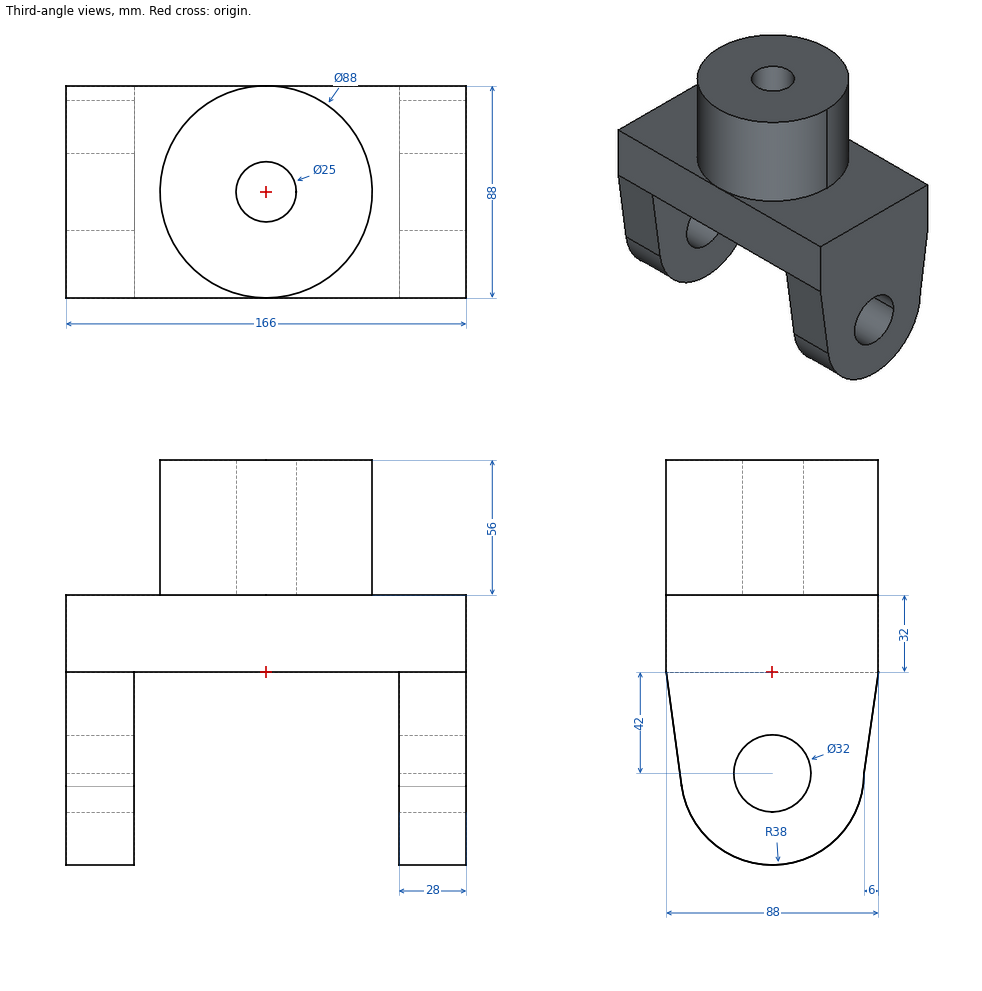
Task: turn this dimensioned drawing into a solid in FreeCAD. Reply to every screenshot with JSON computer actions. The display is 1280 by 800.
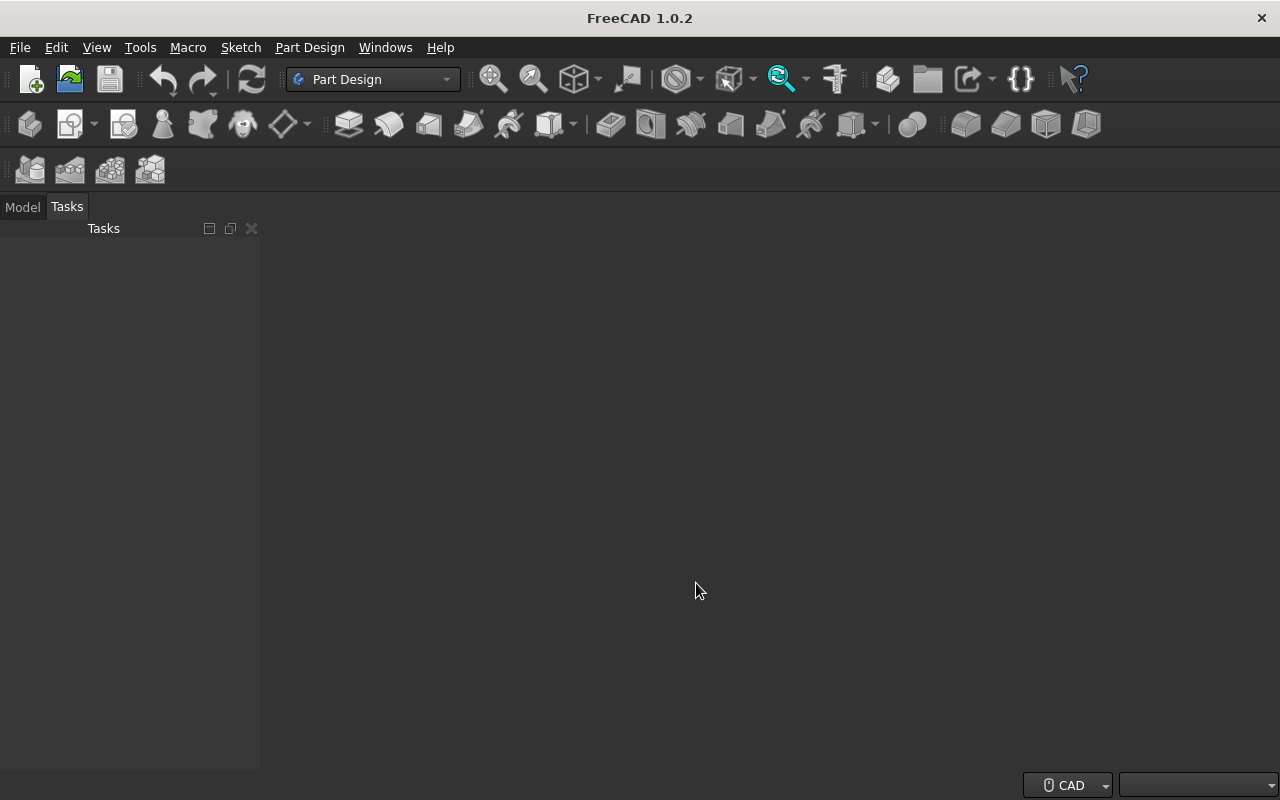
{"action": "left_click", "coordinate": [30, 80]}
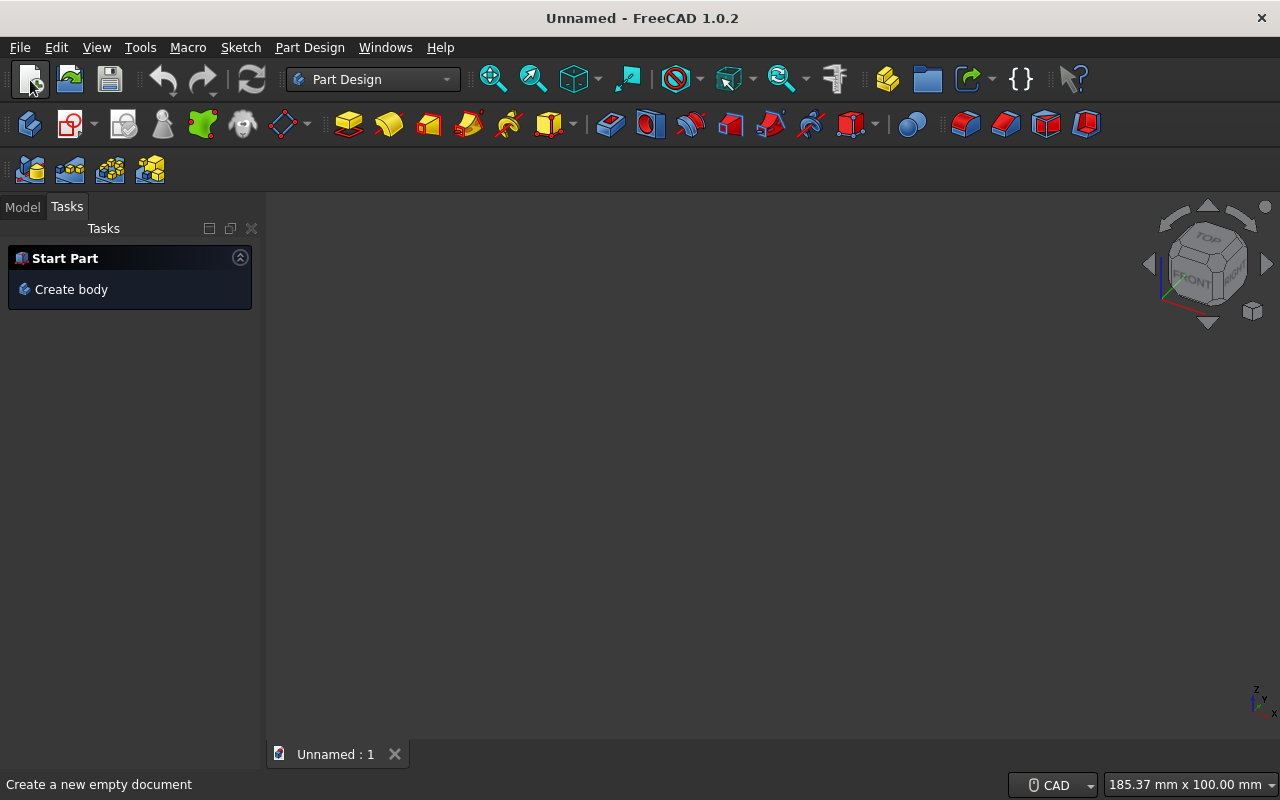
{"action": "left_click", "coordinate": [70, 124]}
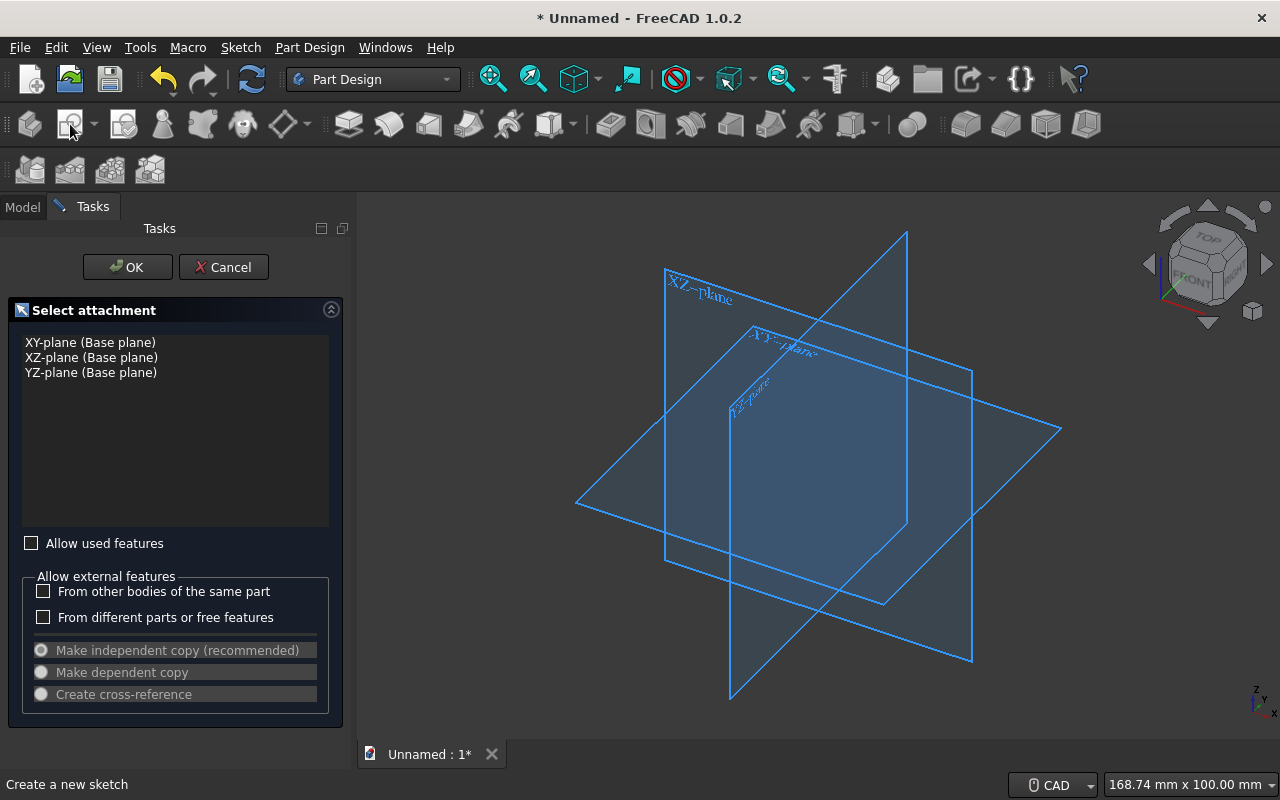
{"action": "left_click", "coordinate": [82, 342]}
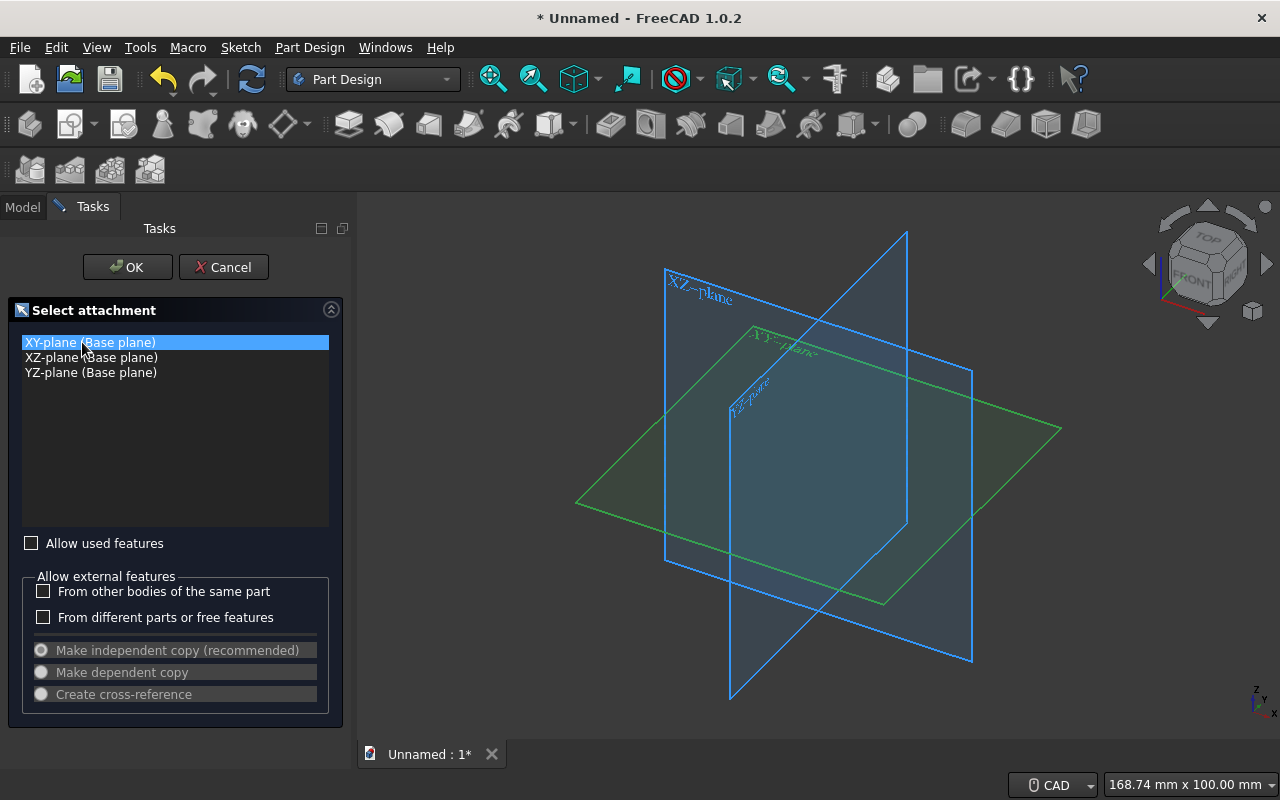
{"action": "left_click", "coordinate": [128, 267]}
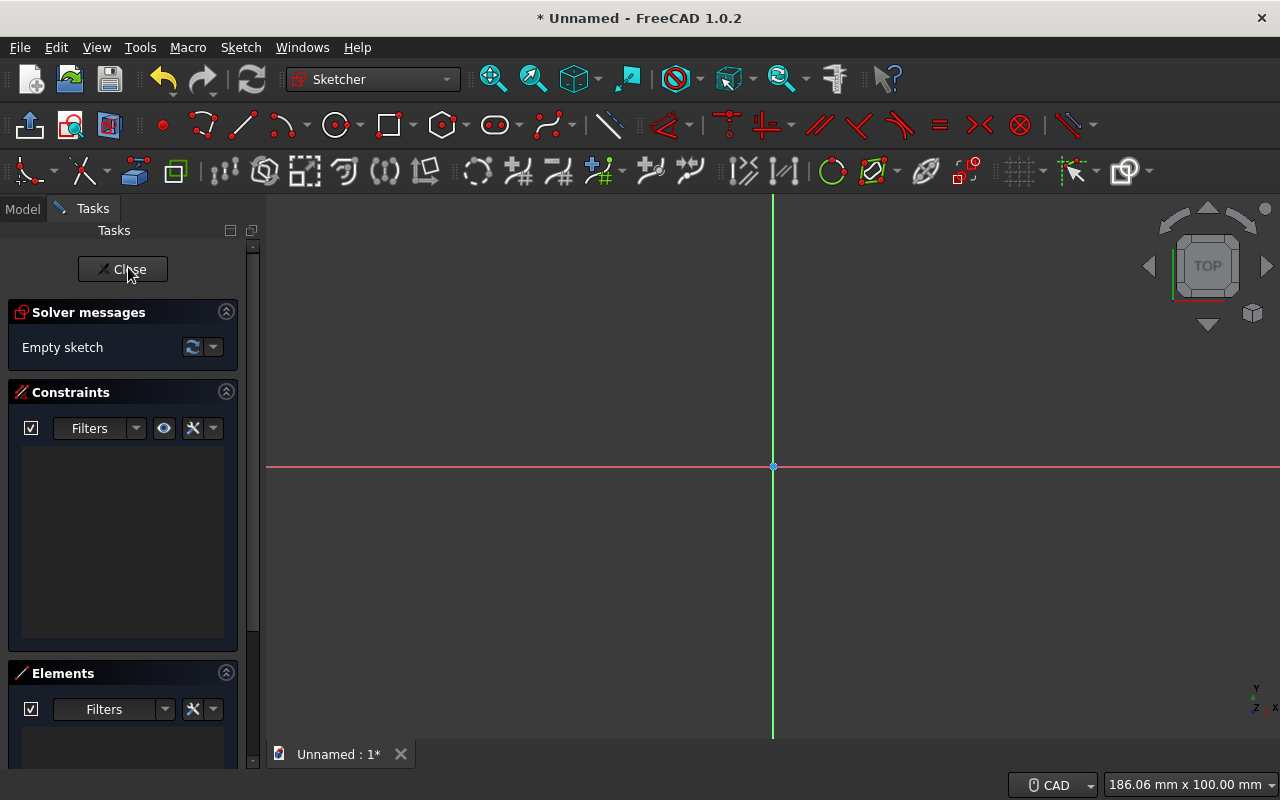
{"action": "scroll", "coordinate": [565, 466], "scroll_direction": "down", "scroll_amount": 2}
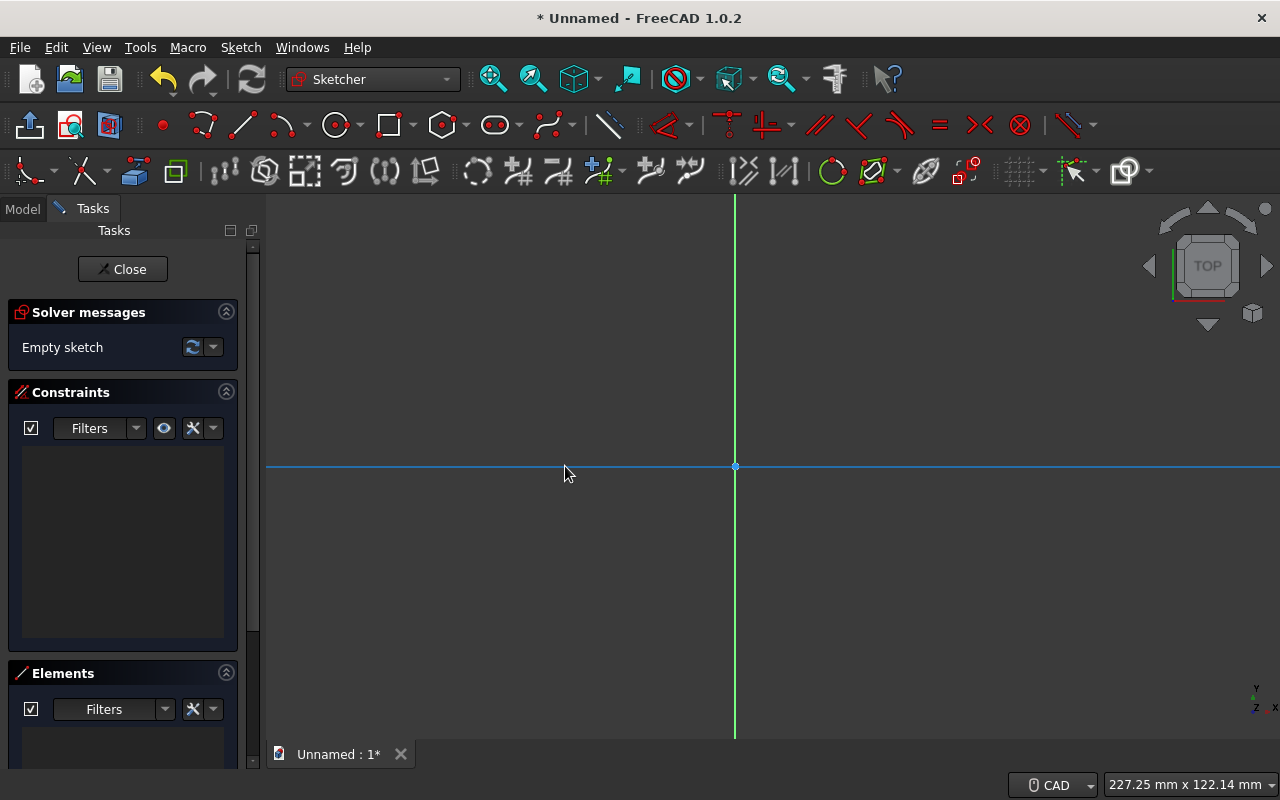
{"action": "key", "text": "g v"}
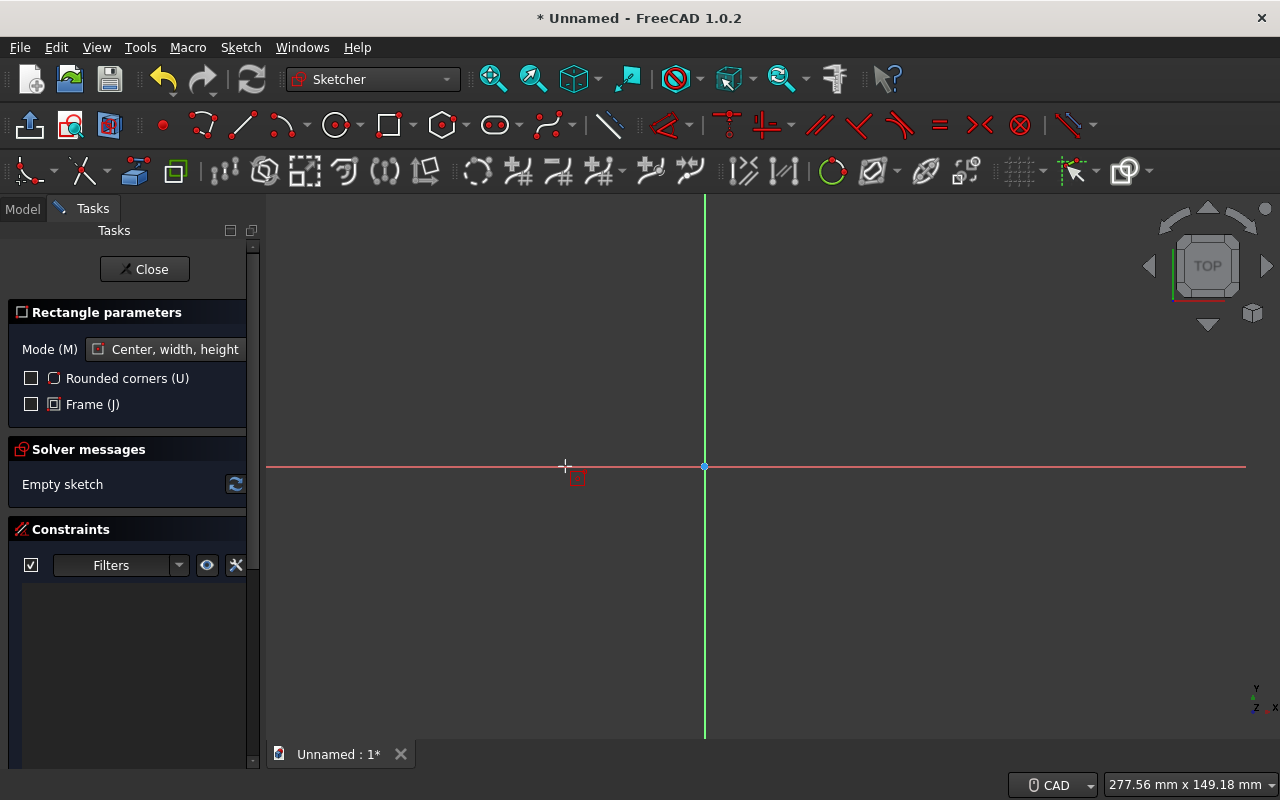
{"action": "left_click", "coordinate": [705, 466]}
{"action": "left_click", "coordinate": [1008, 306]}
{"action": "key", "text": "Escape"}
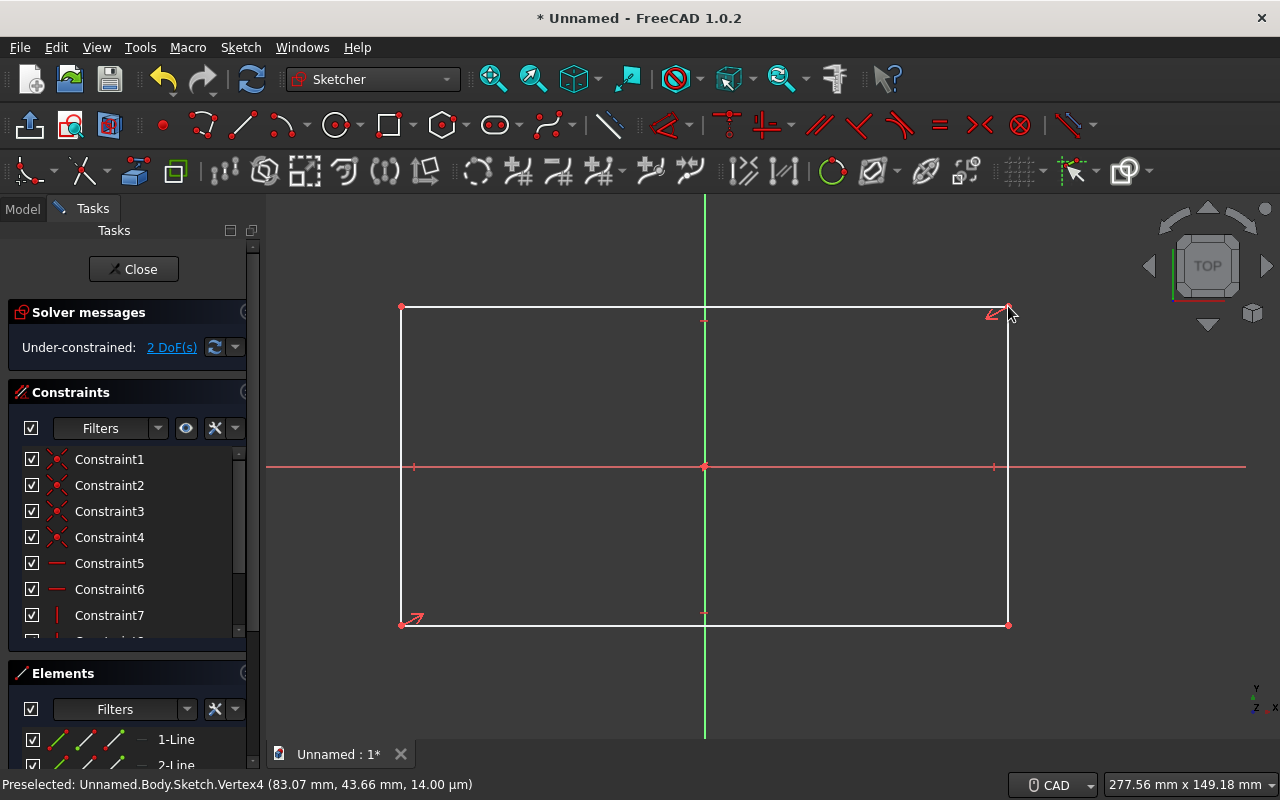
{"action": "left_click", "coordinate": [664, 126]}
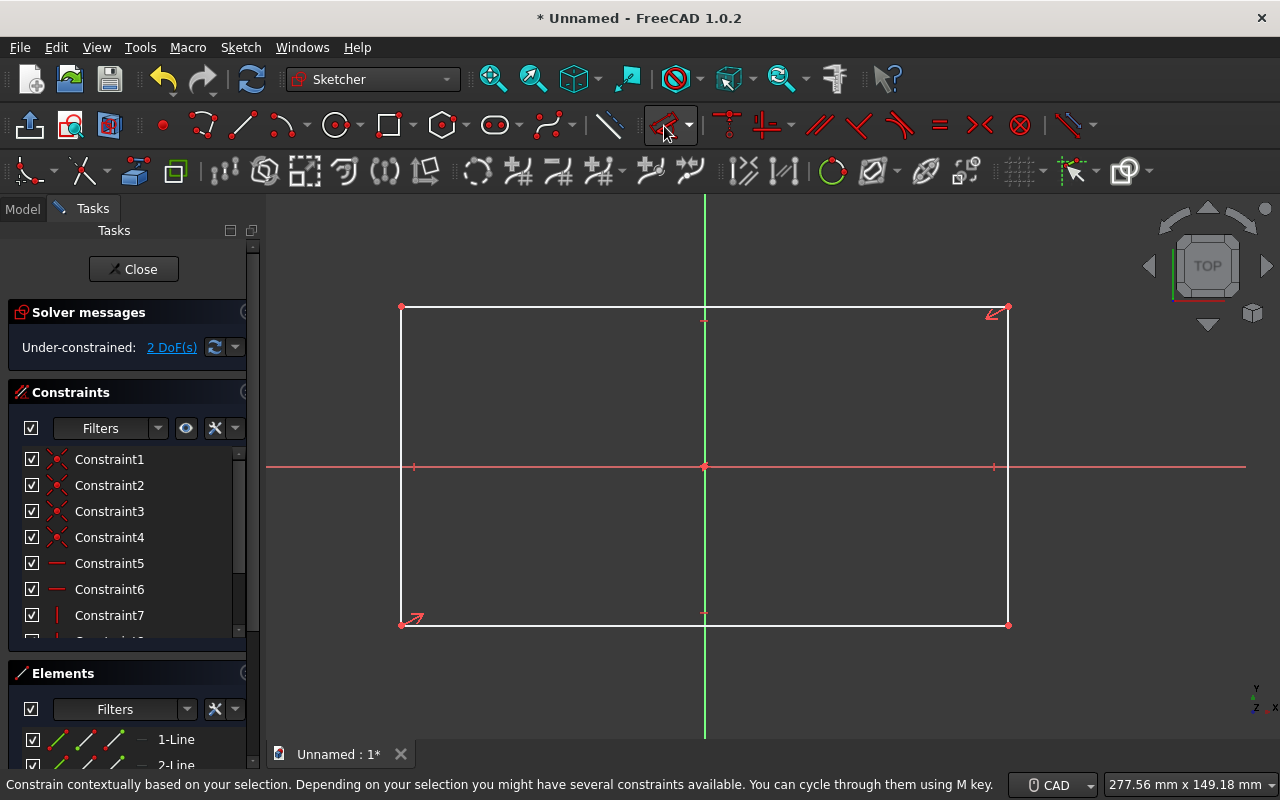
{"action": "left_click", "coordinate": [1008, 530]}
{"action": "left_click", "coordinate": [1042, 393]}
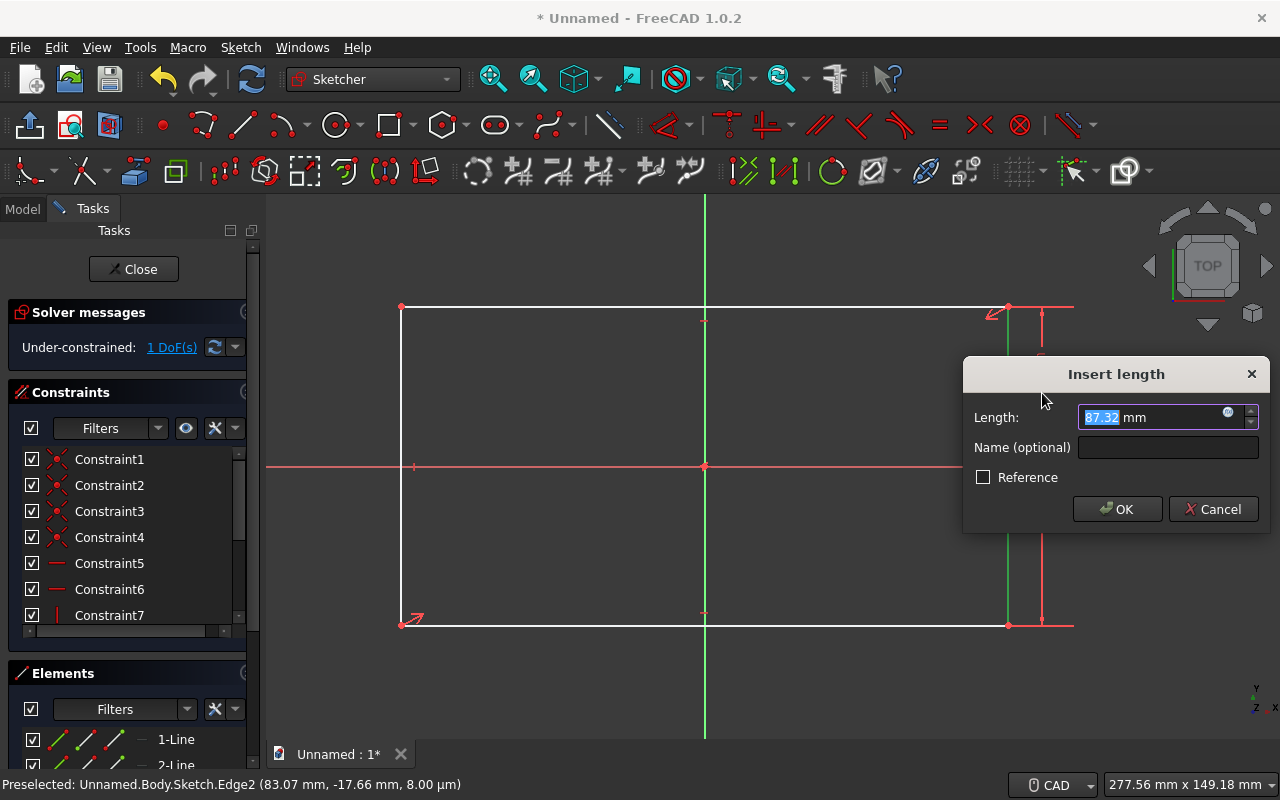
{"action": "type", "text": "88"}
{"action": "key", "text": "Return"}